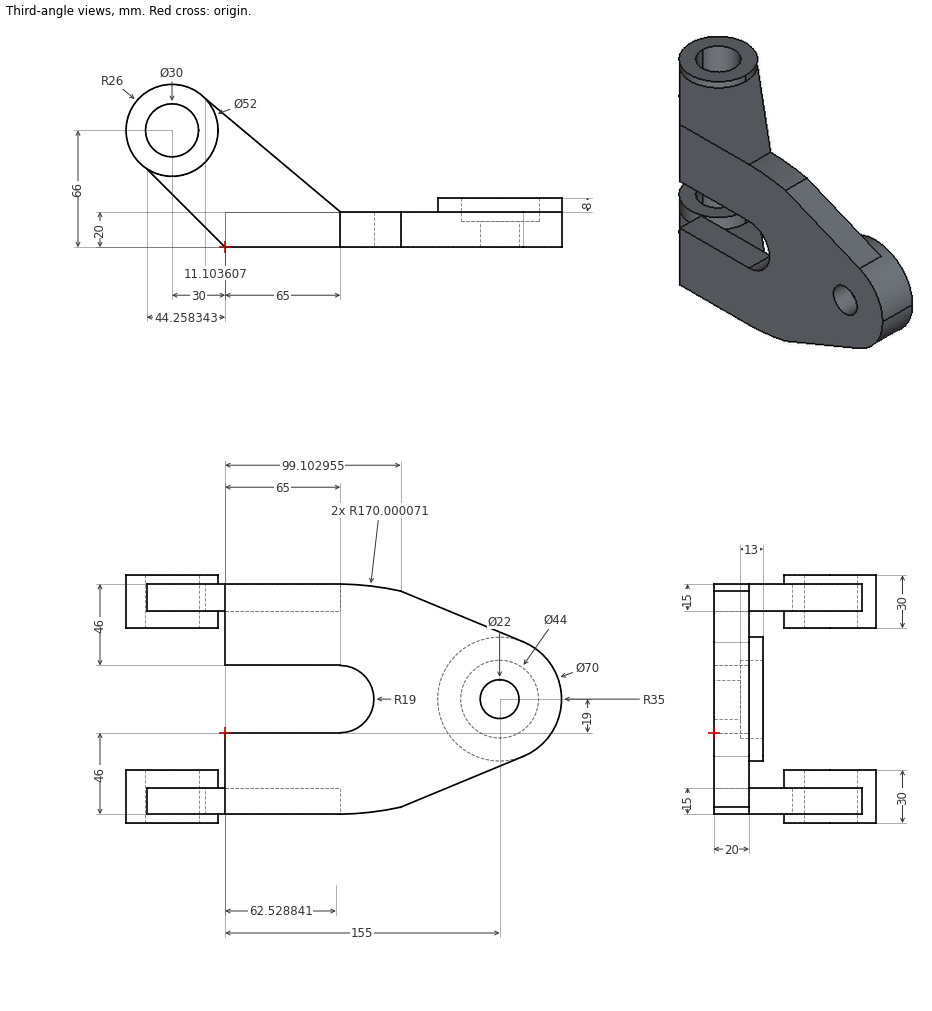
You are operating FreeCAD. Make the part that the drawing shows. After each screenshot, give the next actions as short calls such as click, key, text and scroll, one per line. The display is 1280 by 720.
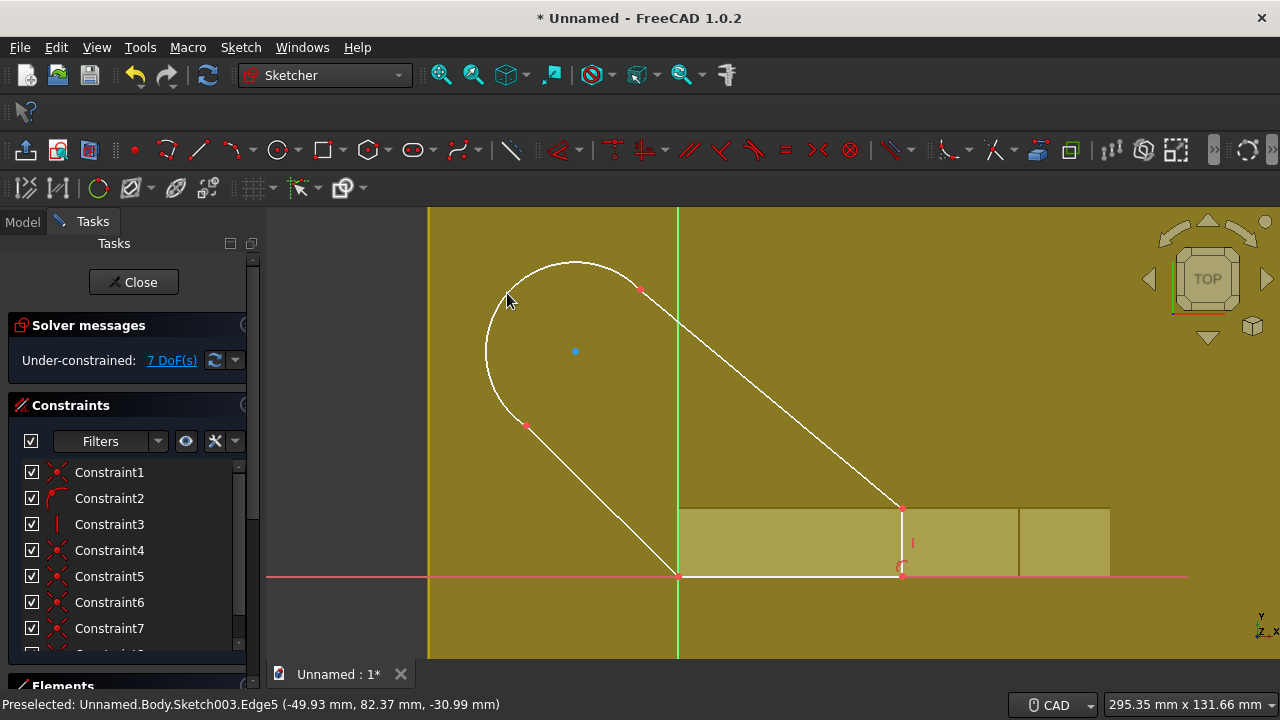
key(d)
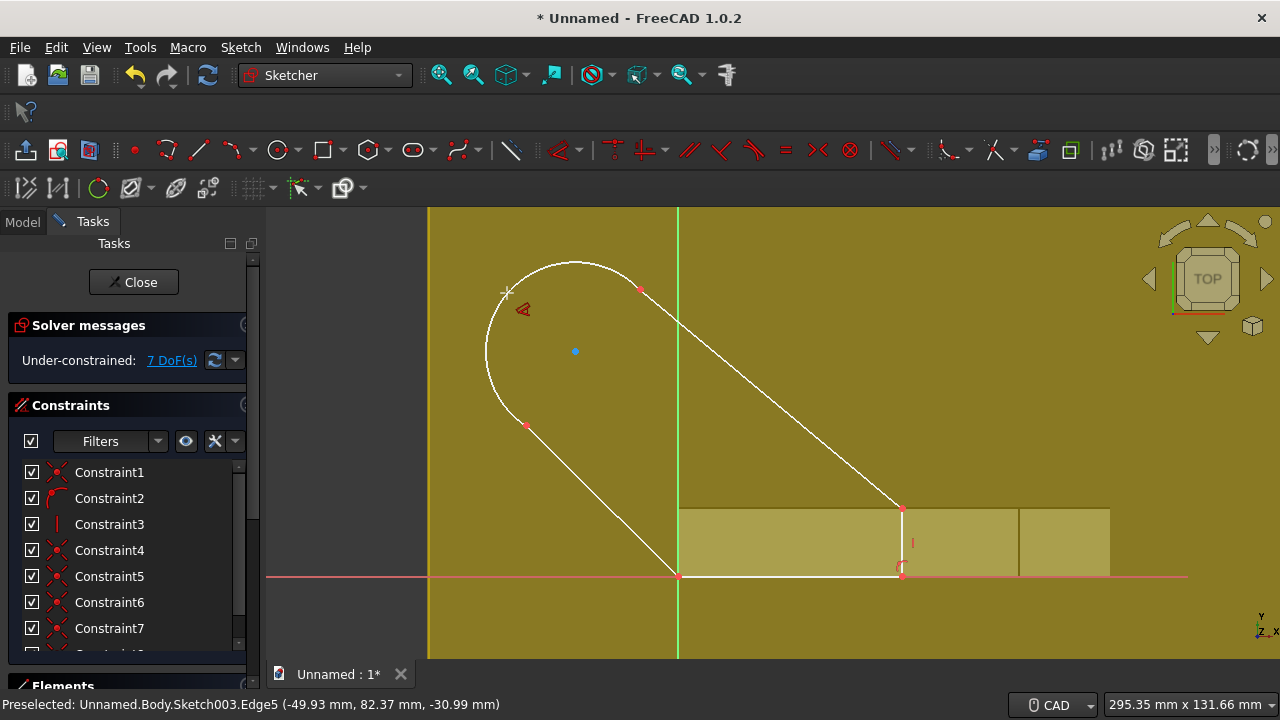
click(558, 264)
click(612, 236)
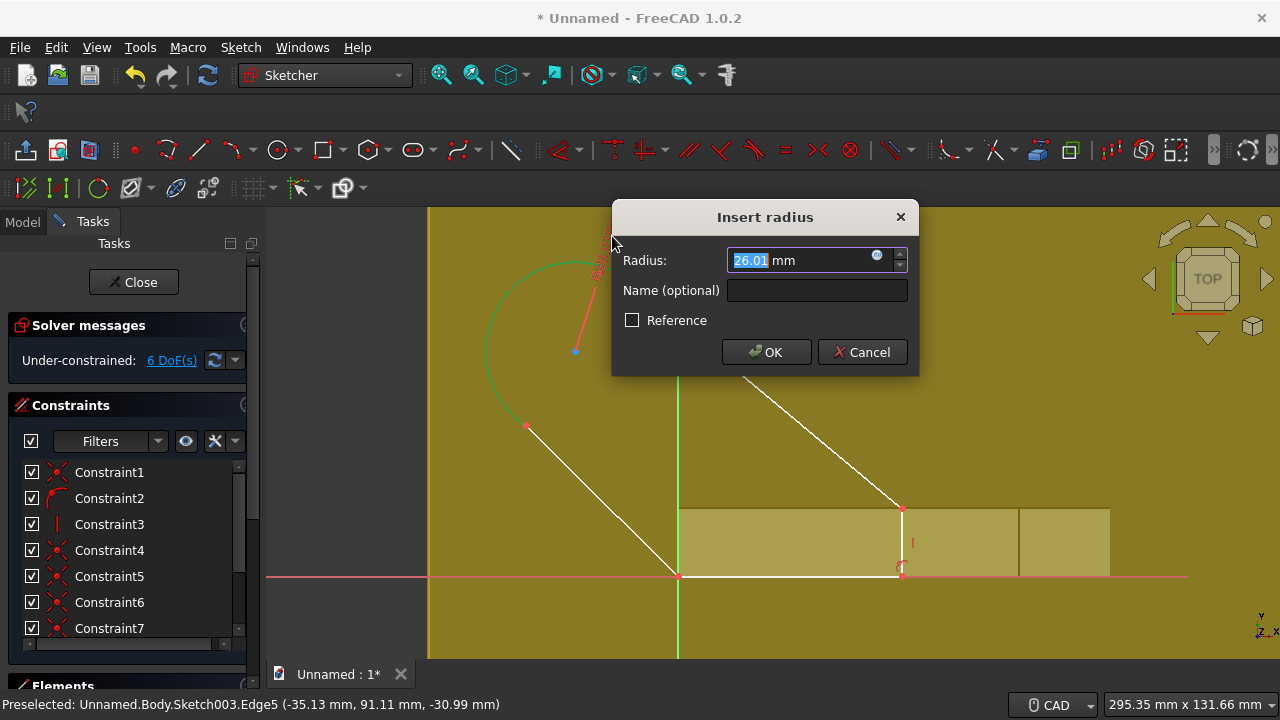
text(26)
key(Return)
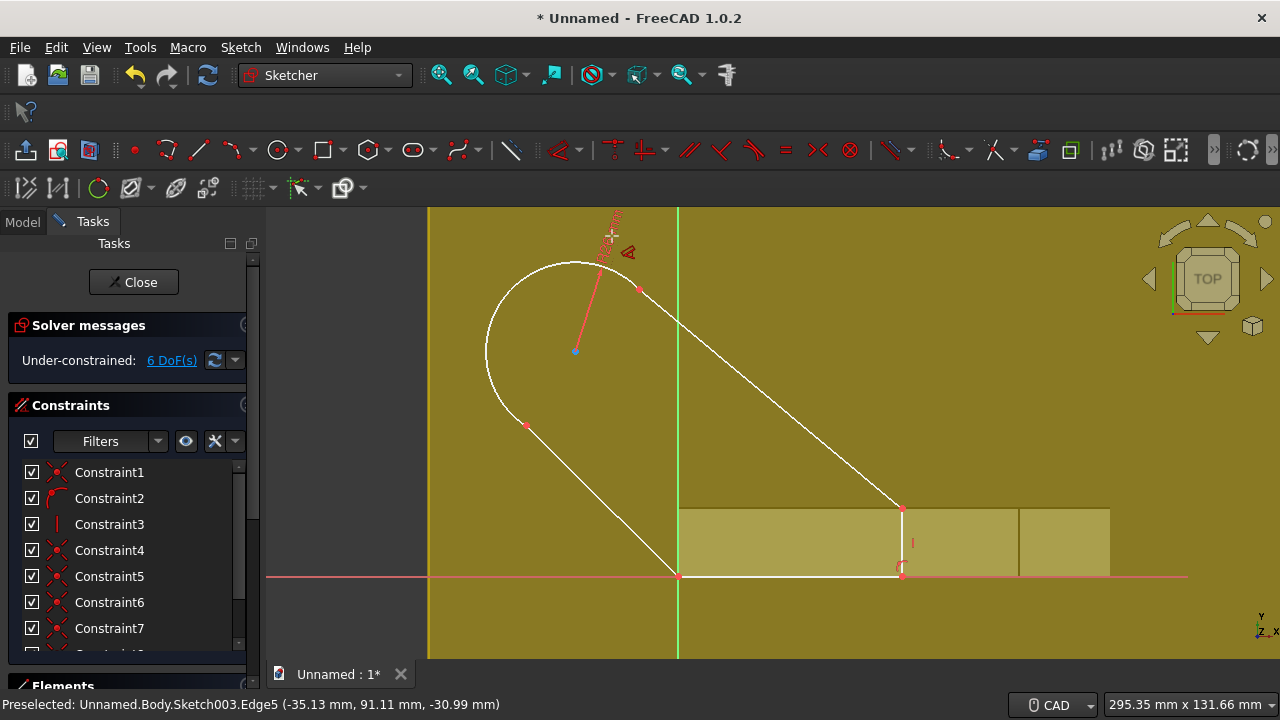
click(902, 529)
click(936, 543)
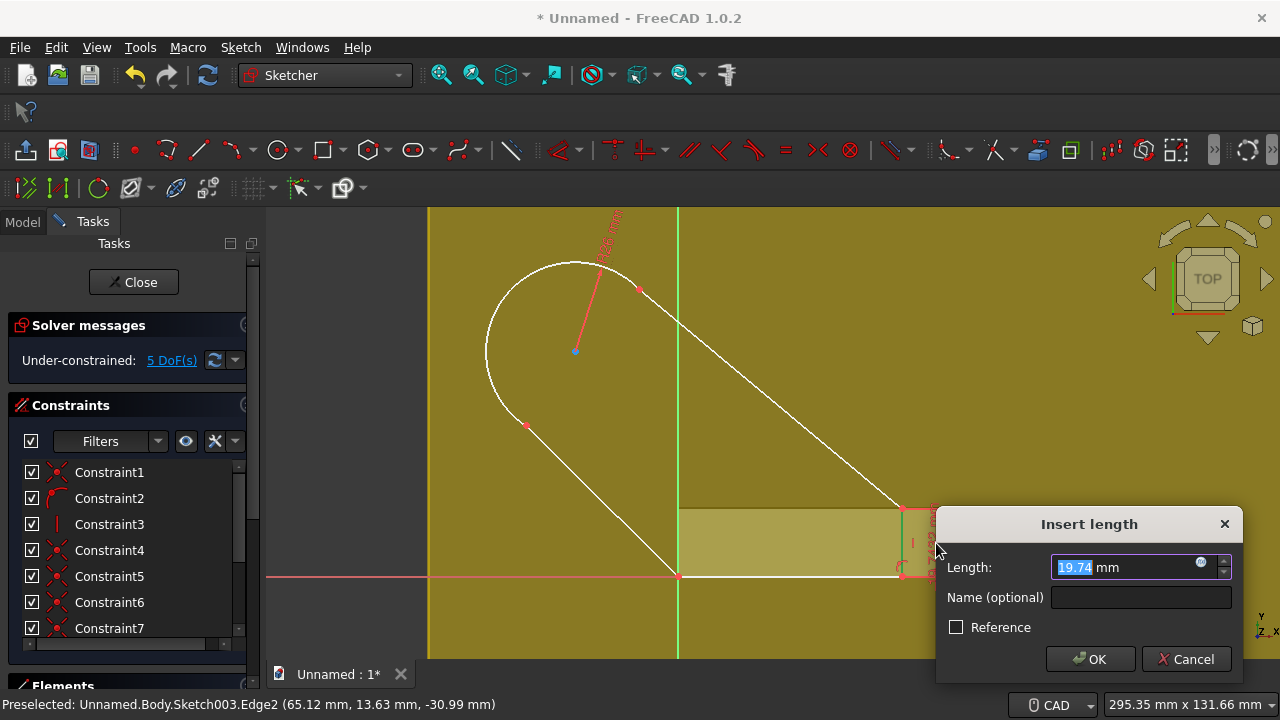
text(20)
key(Return)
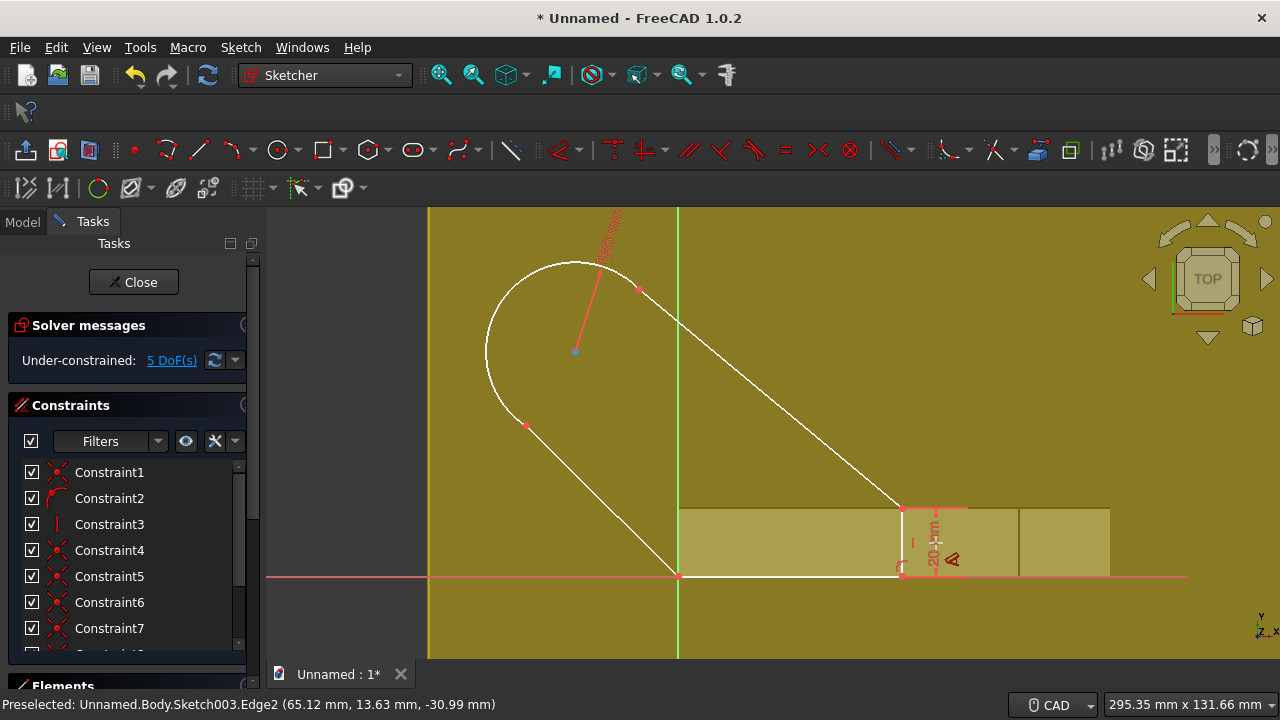
click(835, 577)
click(790, 611)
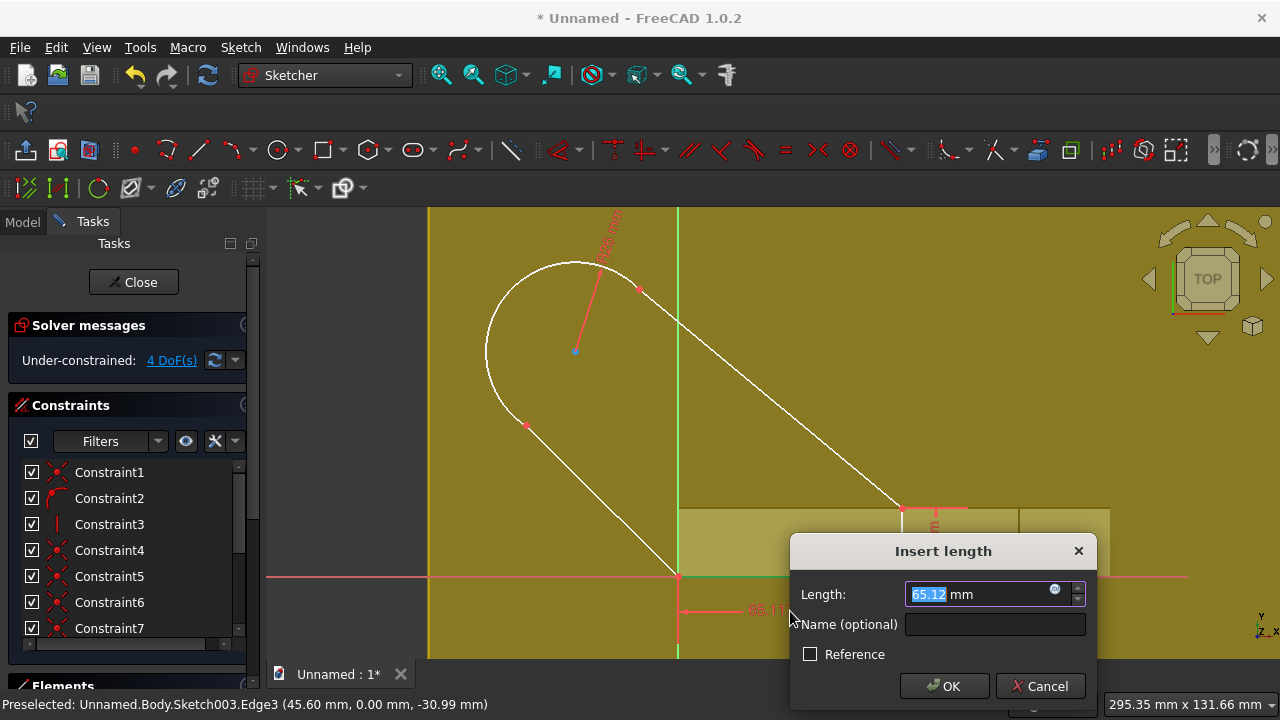
text(65)
key(Return)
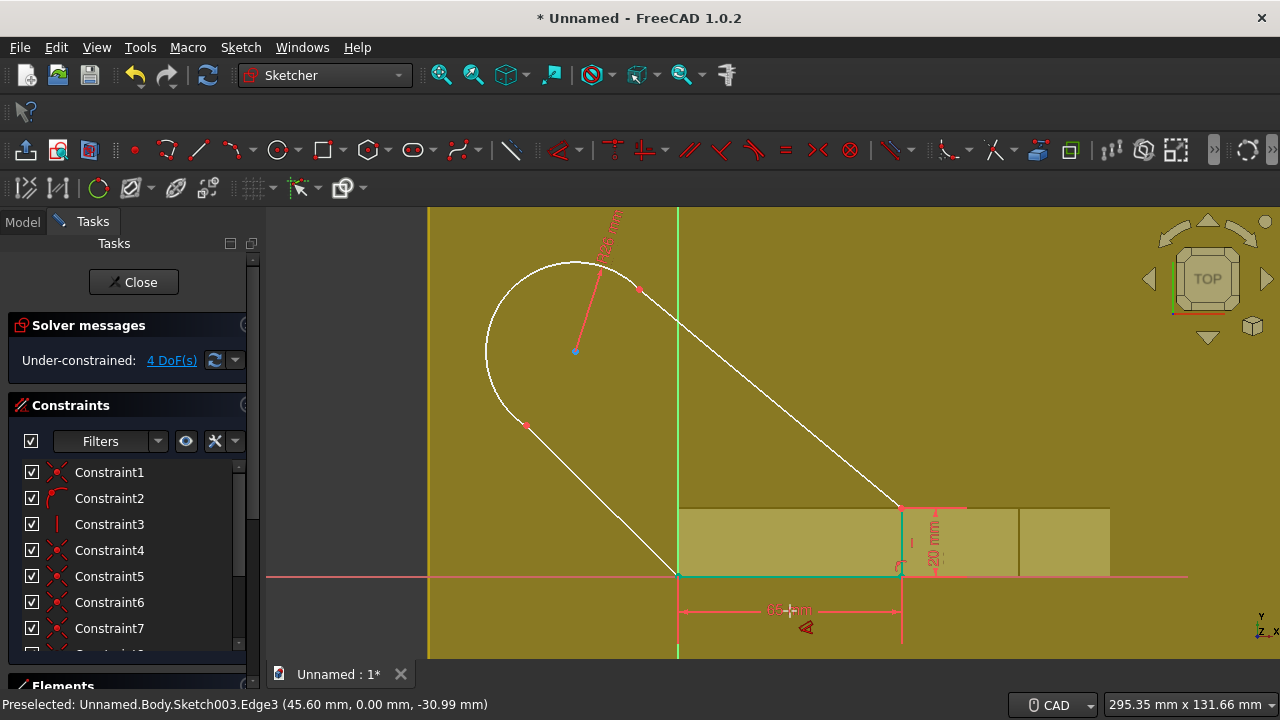
click(575, 352)
click(627, 611)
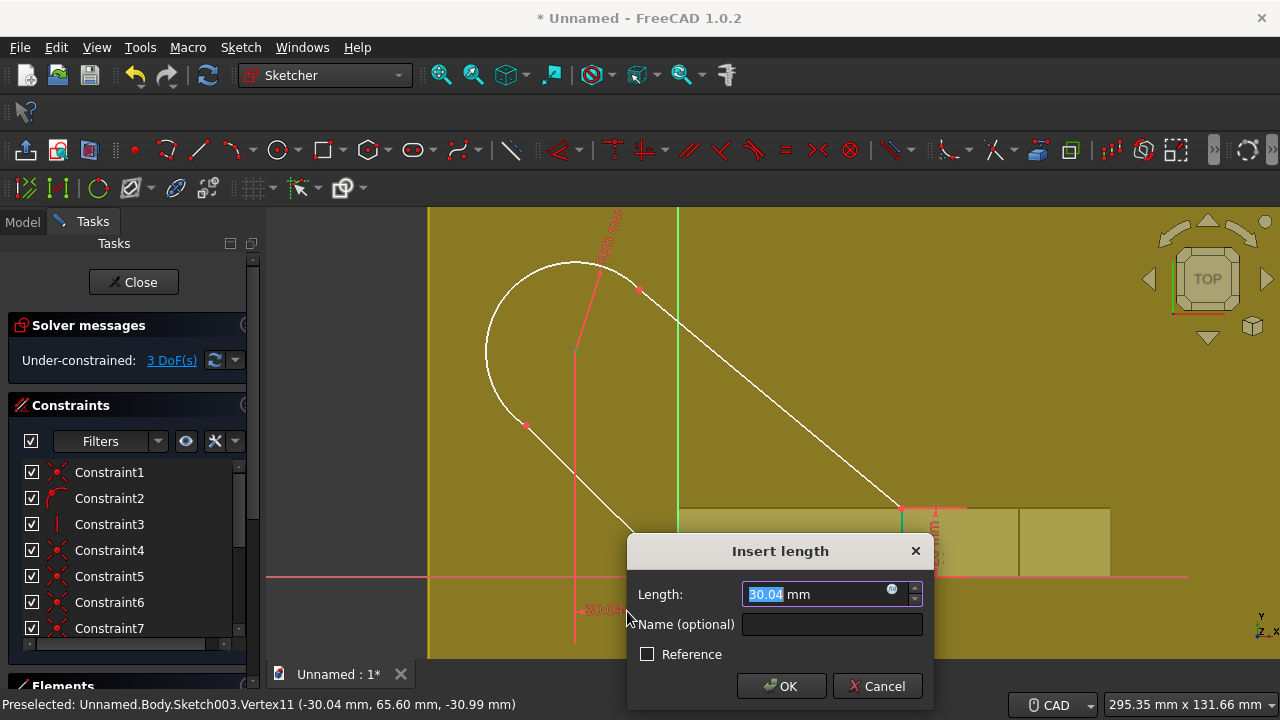
text(30)
key(Return)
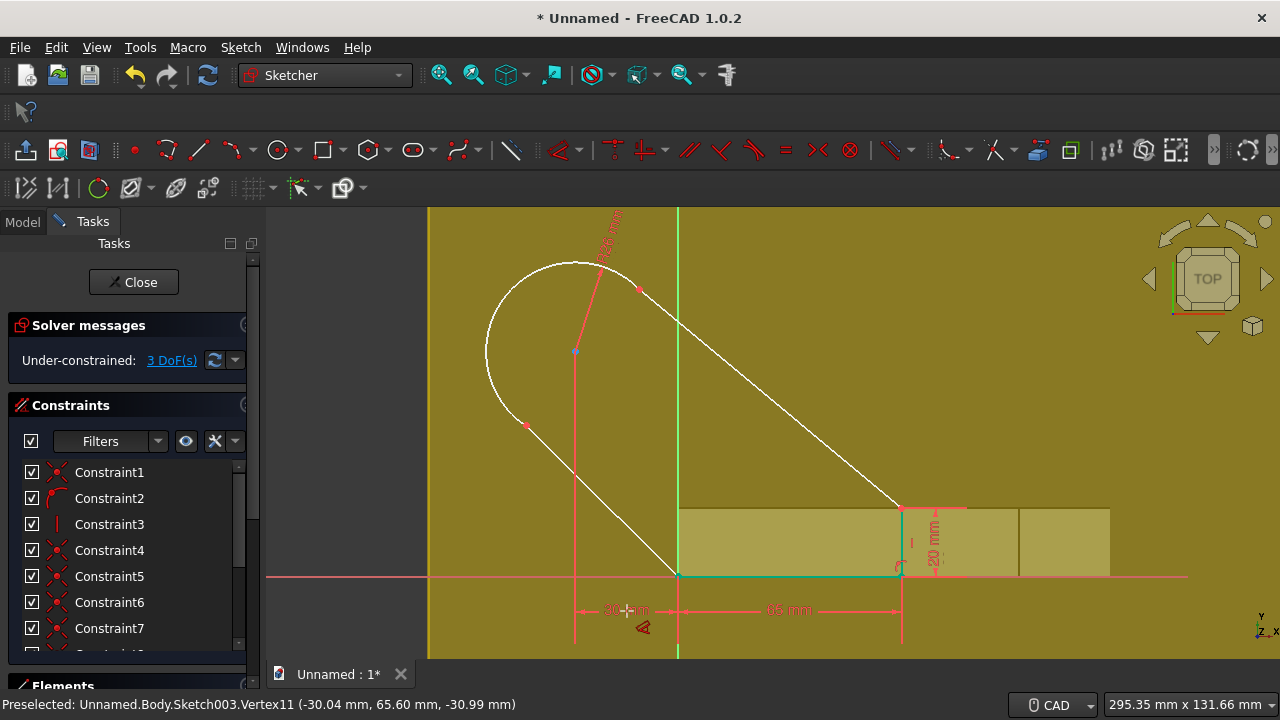
click(575, 352)
click(541, 464)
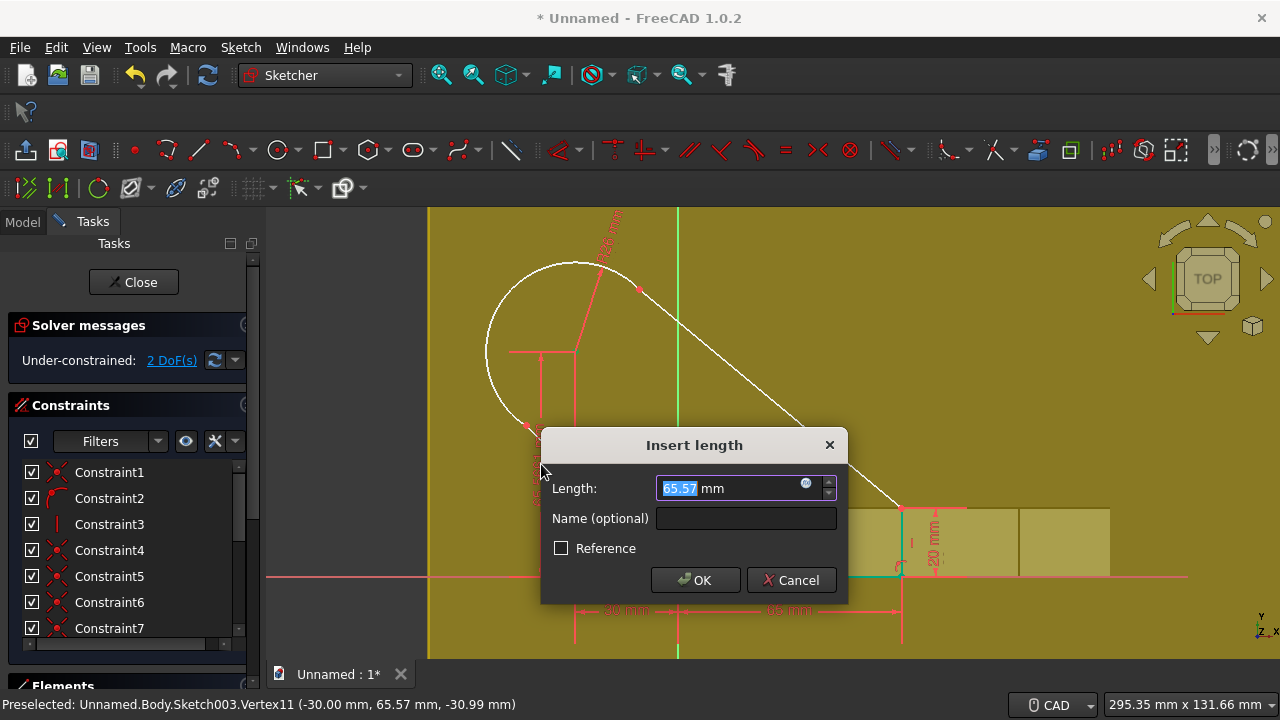
text(66)
key(Return)